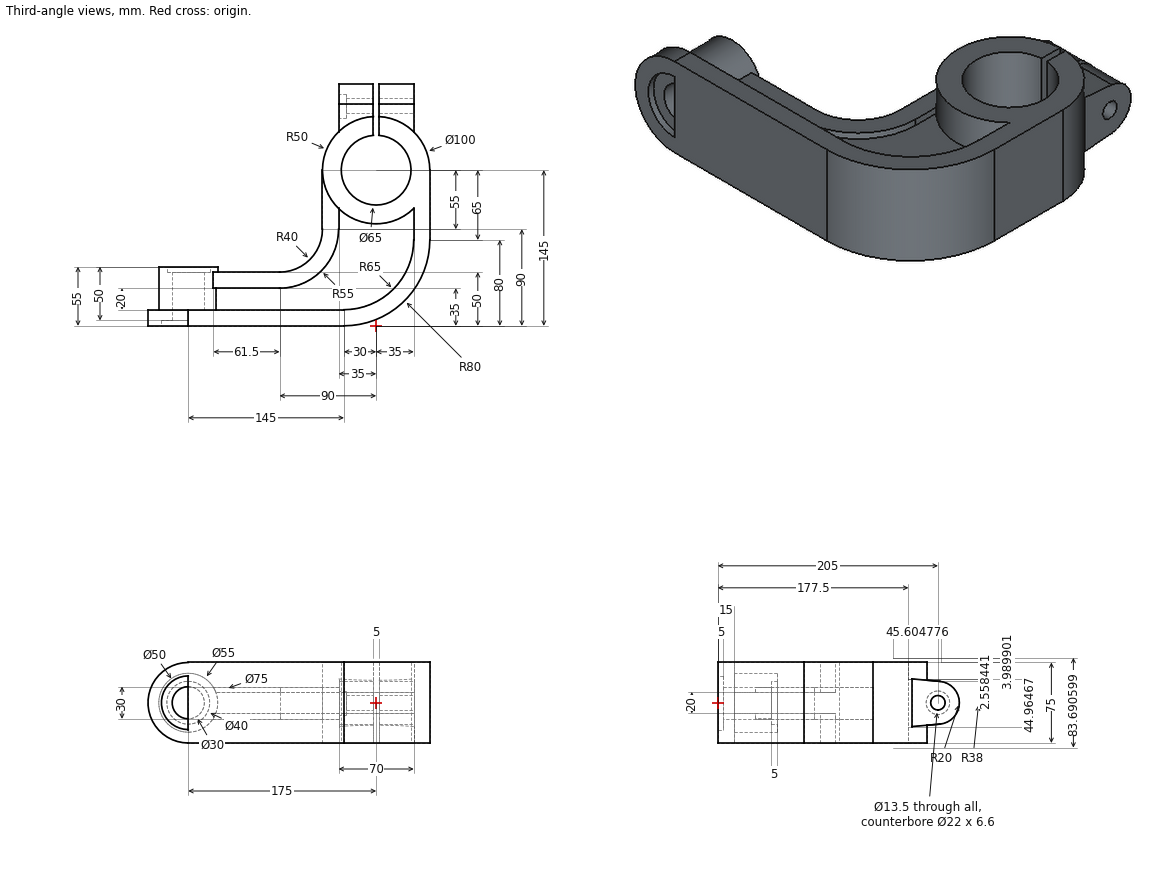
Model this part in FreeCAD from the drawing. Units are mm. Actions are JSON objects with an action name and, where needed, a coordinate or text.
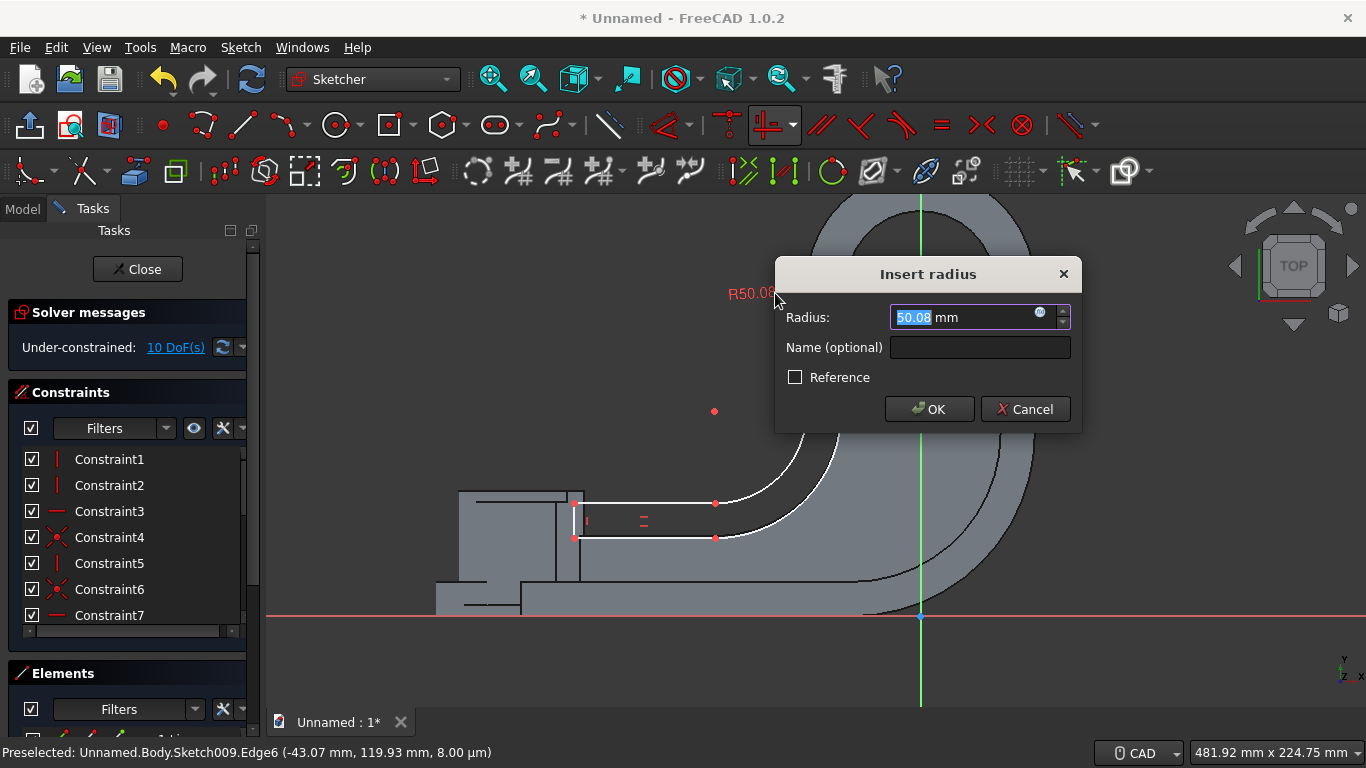
{"action": "type", "text": "50"}
{"action": "key", "text": "Return"}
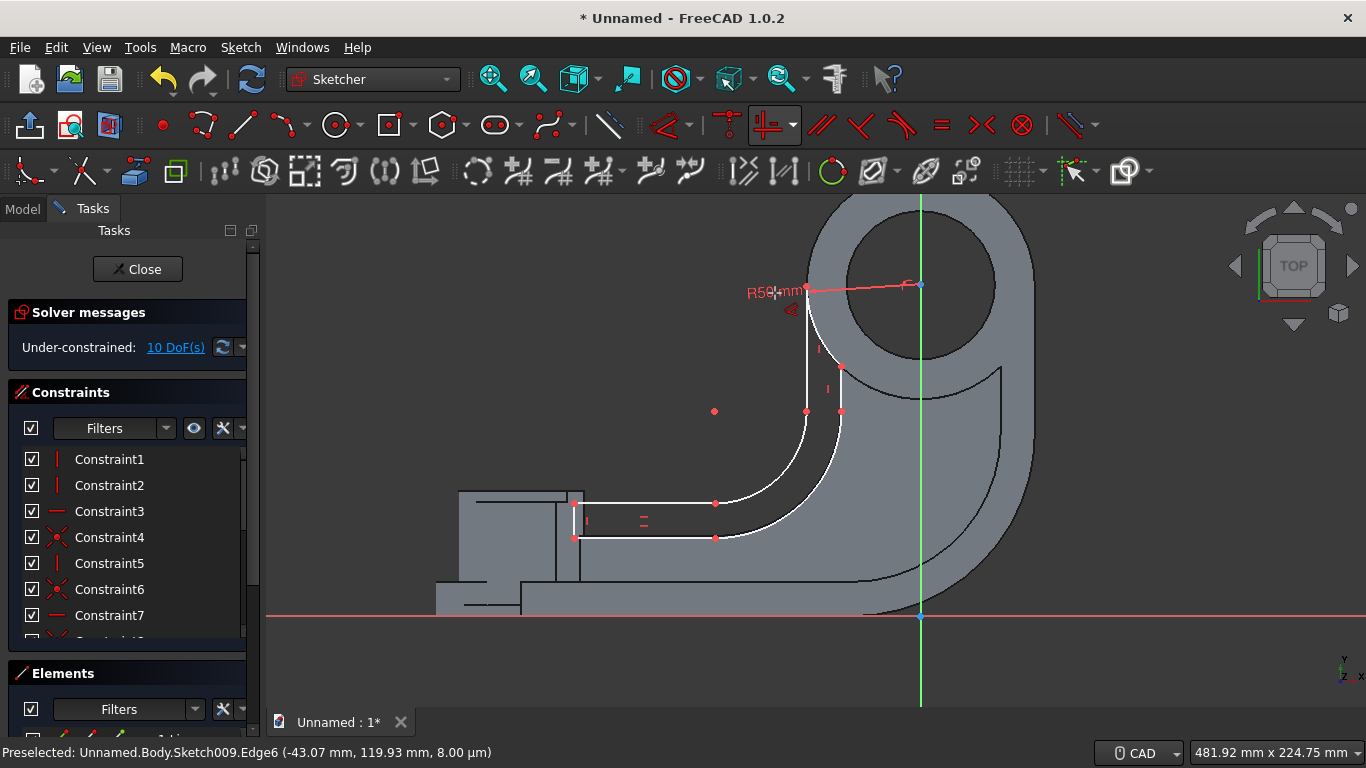
{"action": "left_click", "coordinate": [757, 493]}
{"action": "left_click", "coordinate": [653, 519]}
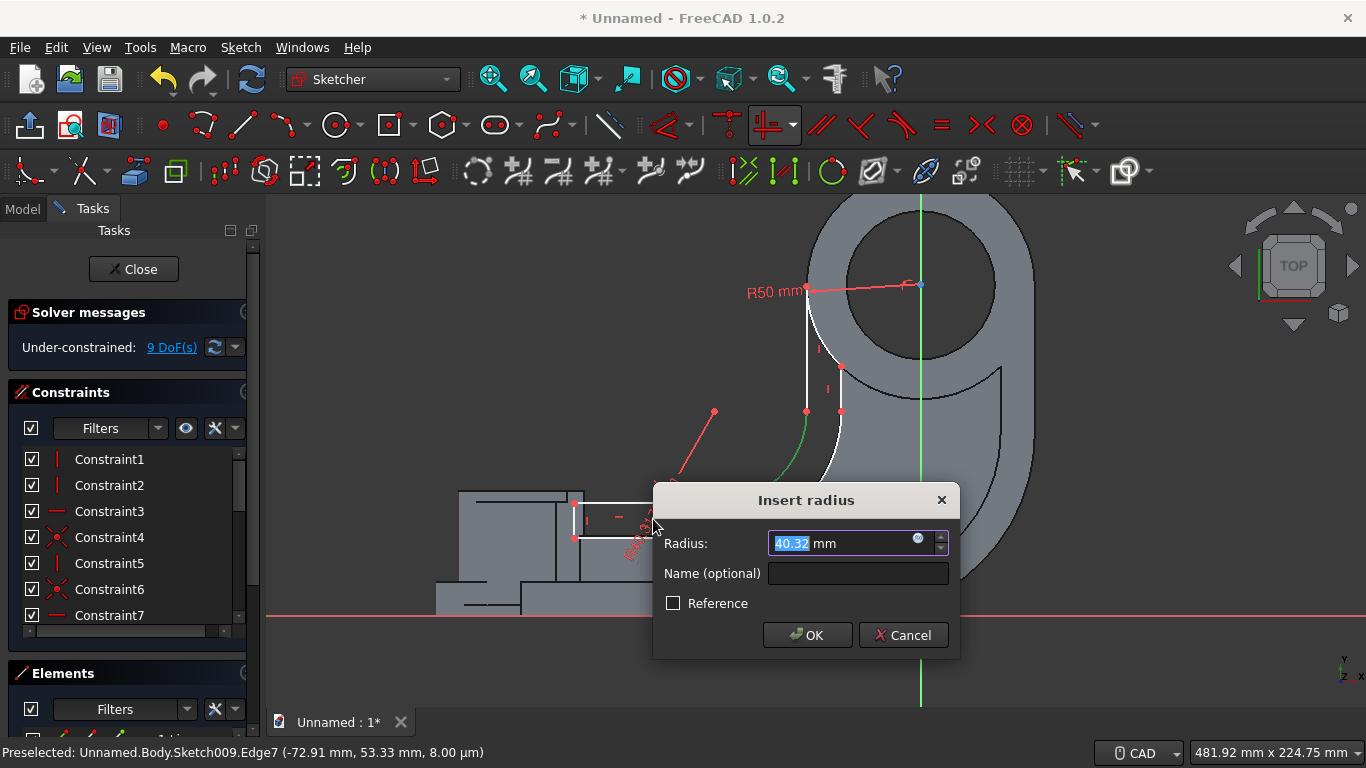
{"action": "type", "text": "40"}
{"action": "key", "text": "Return"}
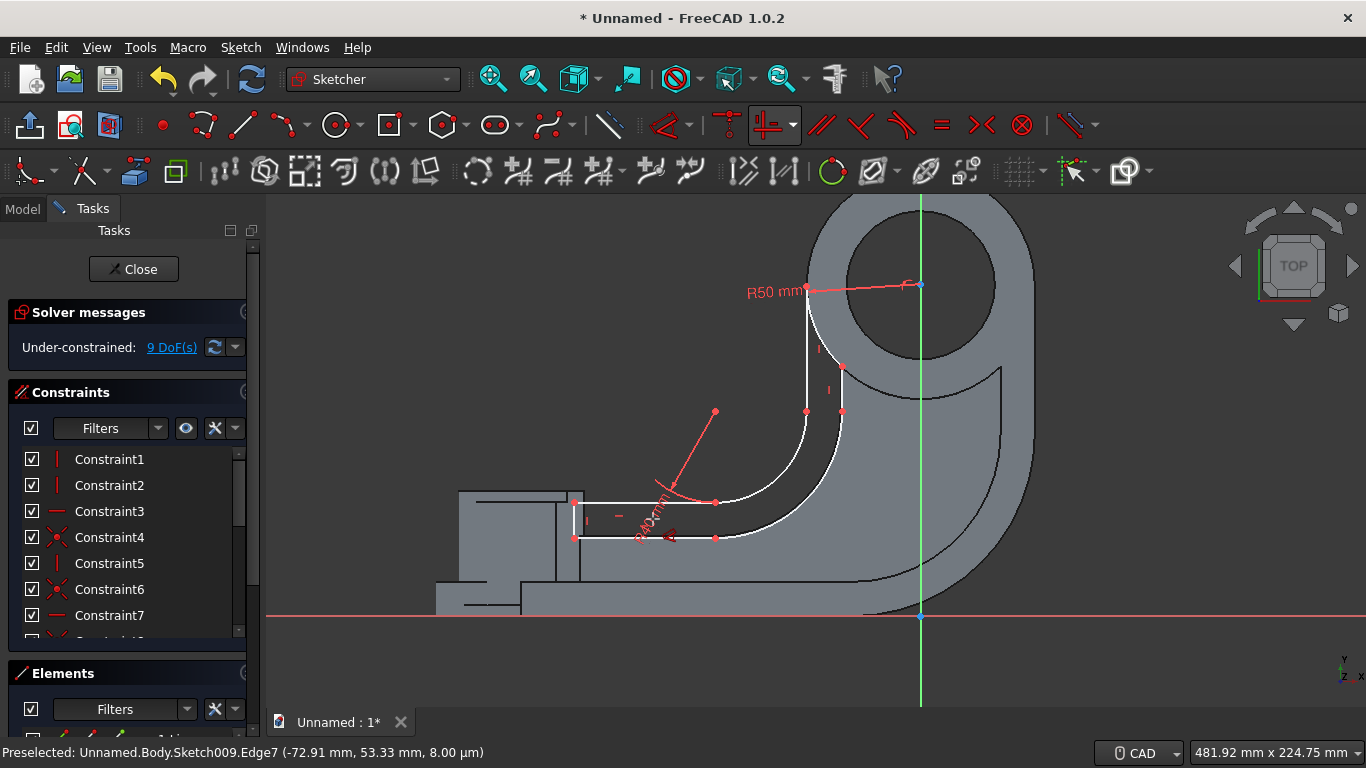
{"action": "left_click", "coordinate": [773, 524]}
{"action": "left_click", "coordinate": [788, 552]}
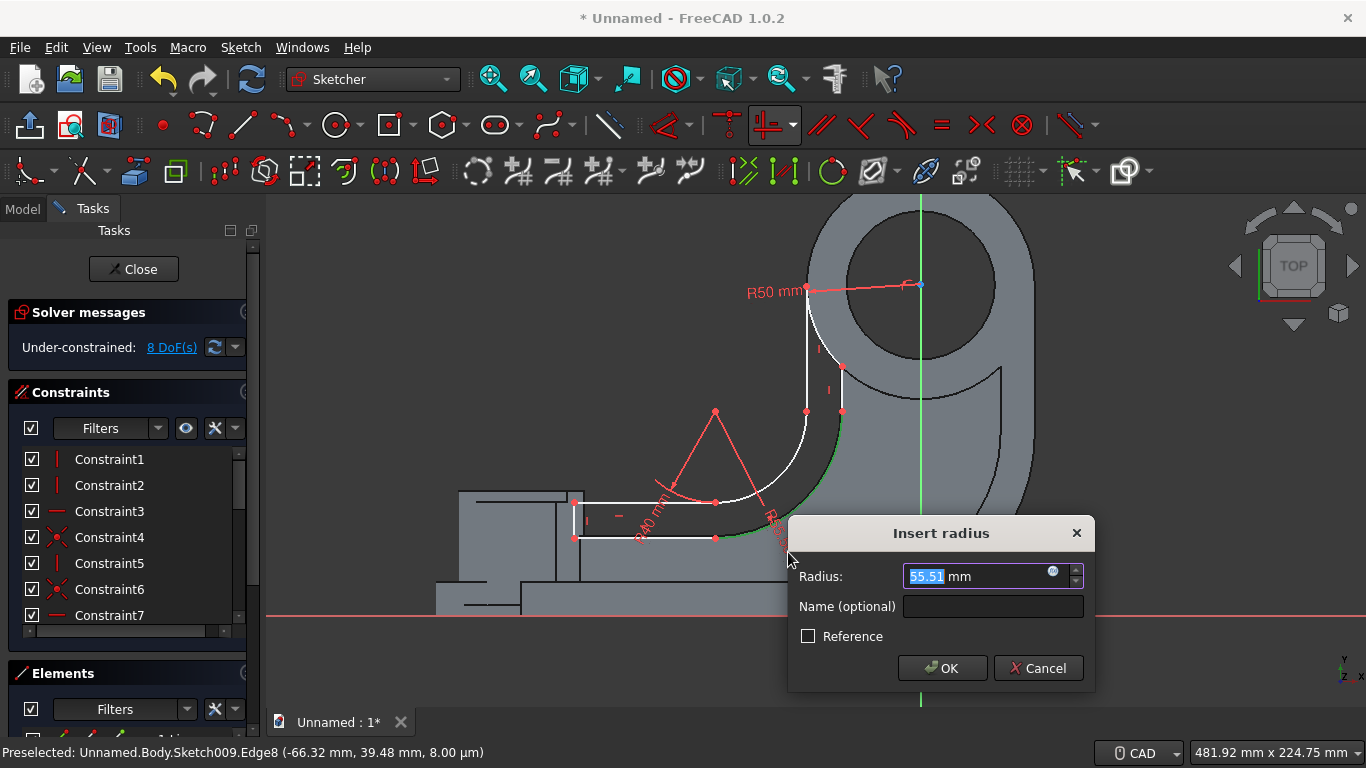
{"action": "type", "text": "55"}
{"action": "key", "text": "Return"}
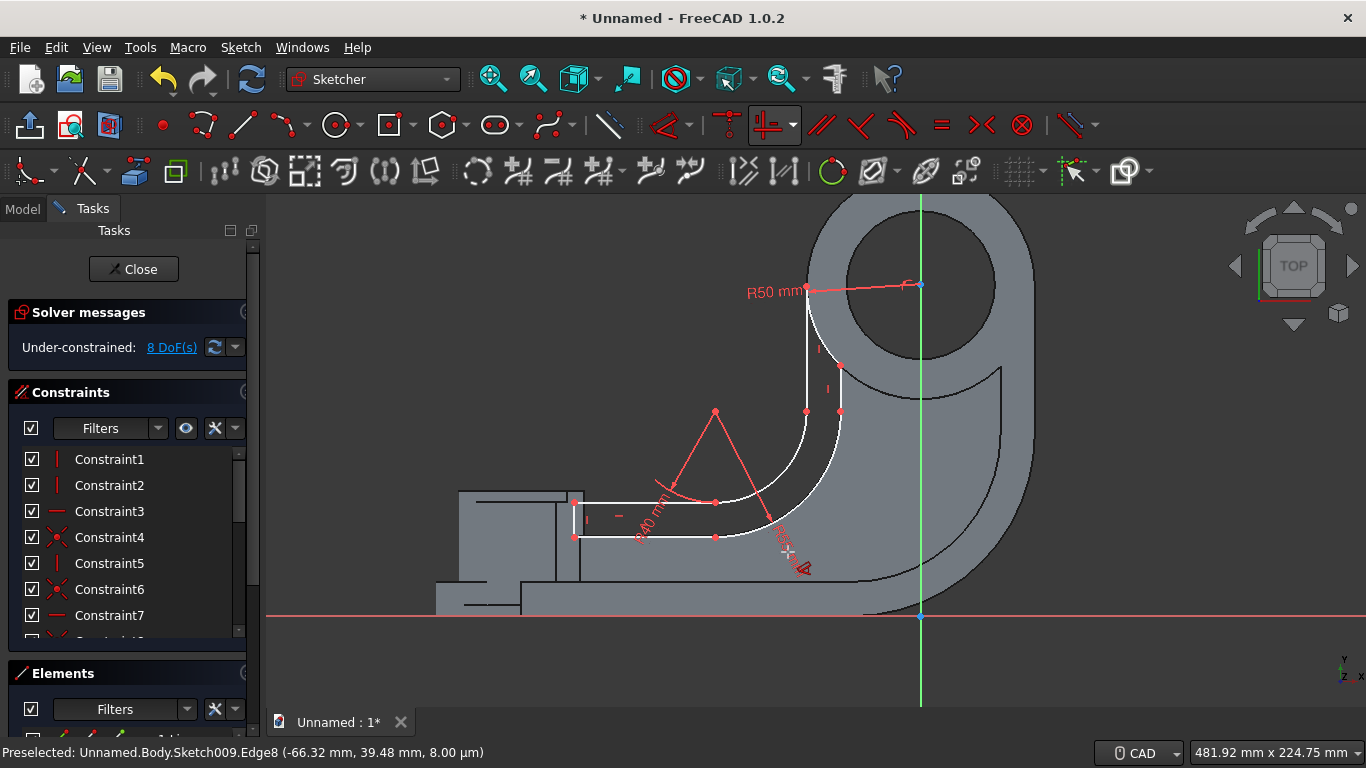
{"action": "left_click", "coordinate": [807, 374]}
{"action": "left_click", "coordinate": [841, 320]}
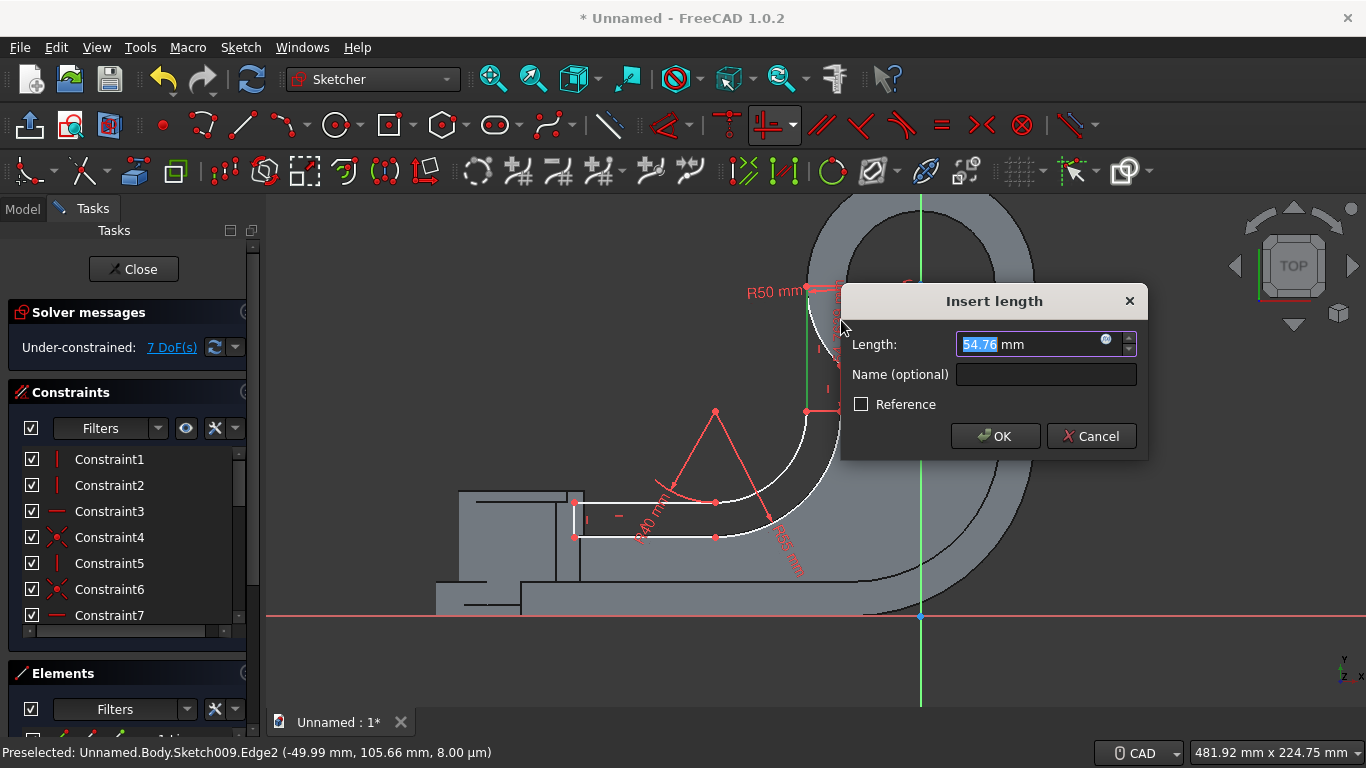
{"action": "type", "text": "55"}
{"action": "key", "text": "Return"}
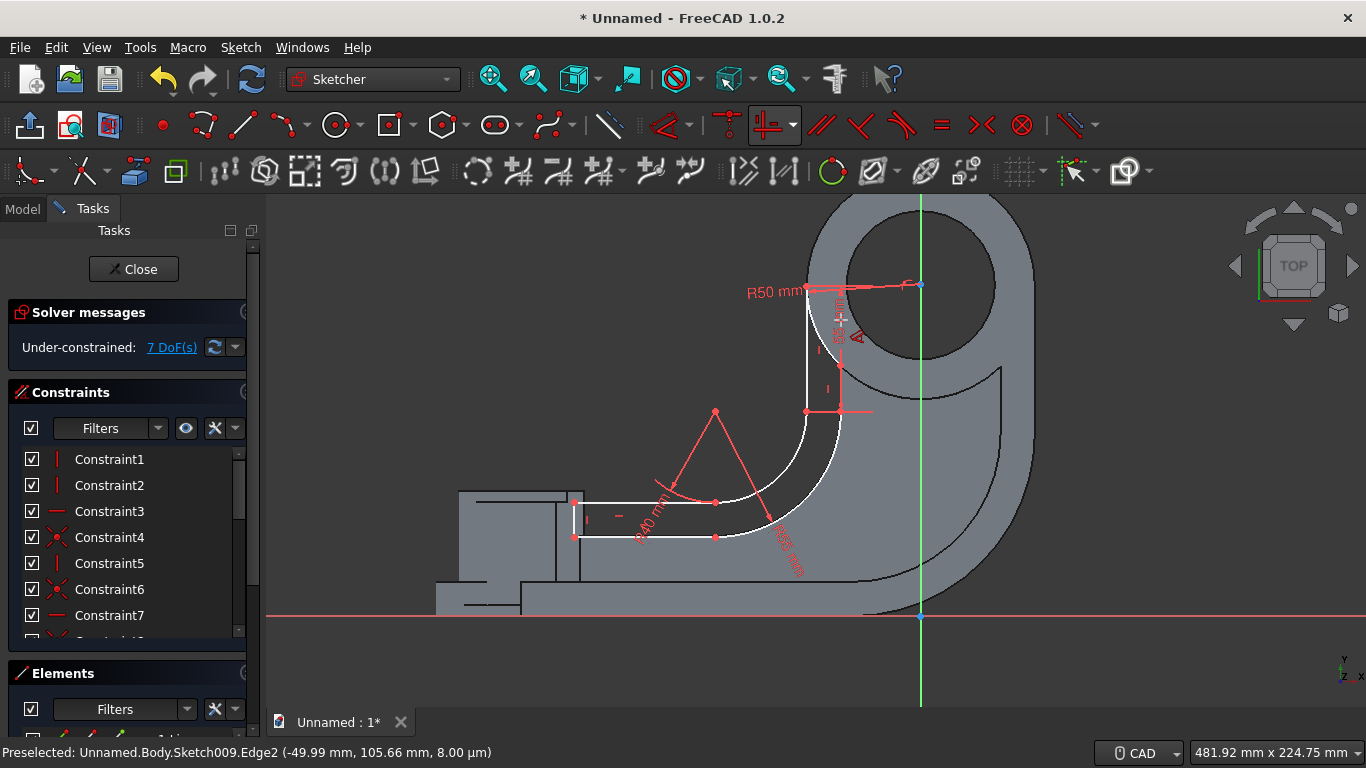
{"action": "left_click", "coordinate": [841, 411]}
{"action": "left_click", "coordinate": [955, 514]}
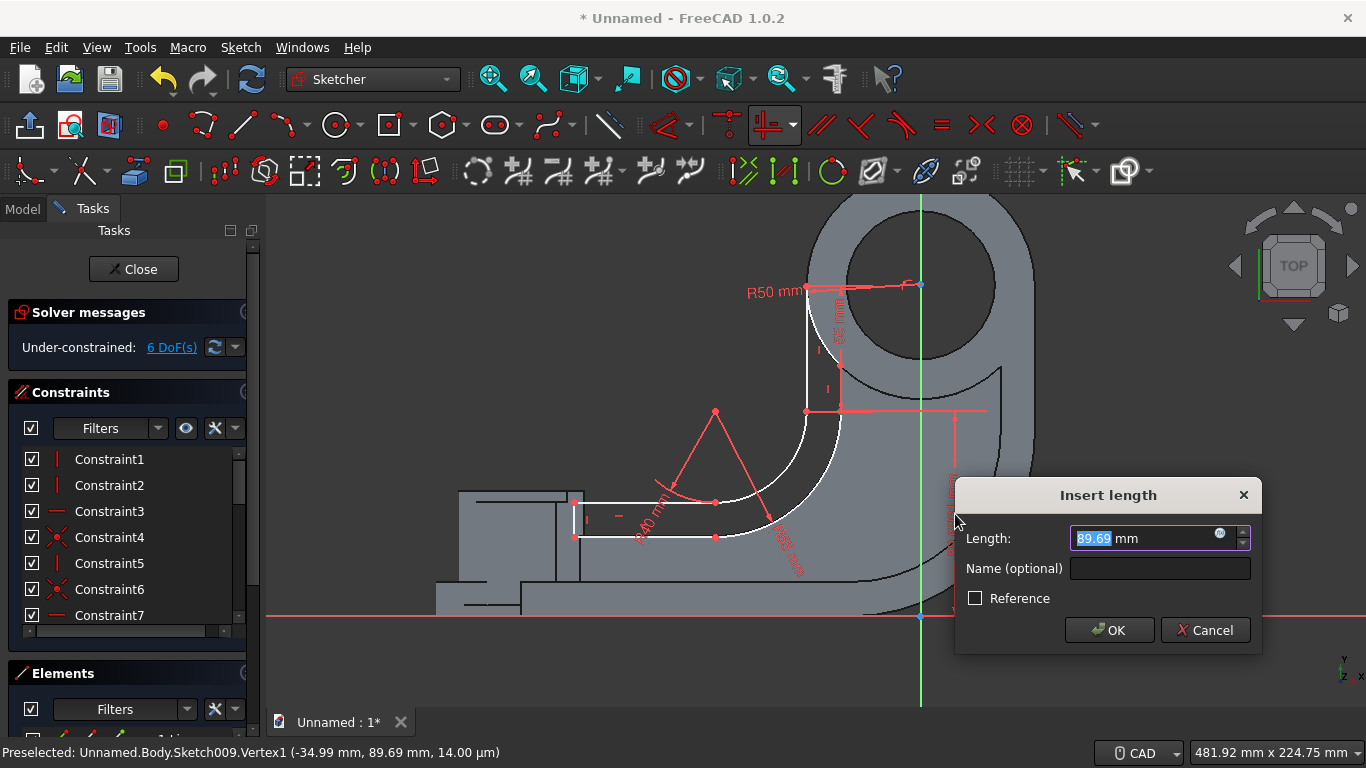
{"action": "type", "text": "90"}
{"action": "key", "text": "Return"}